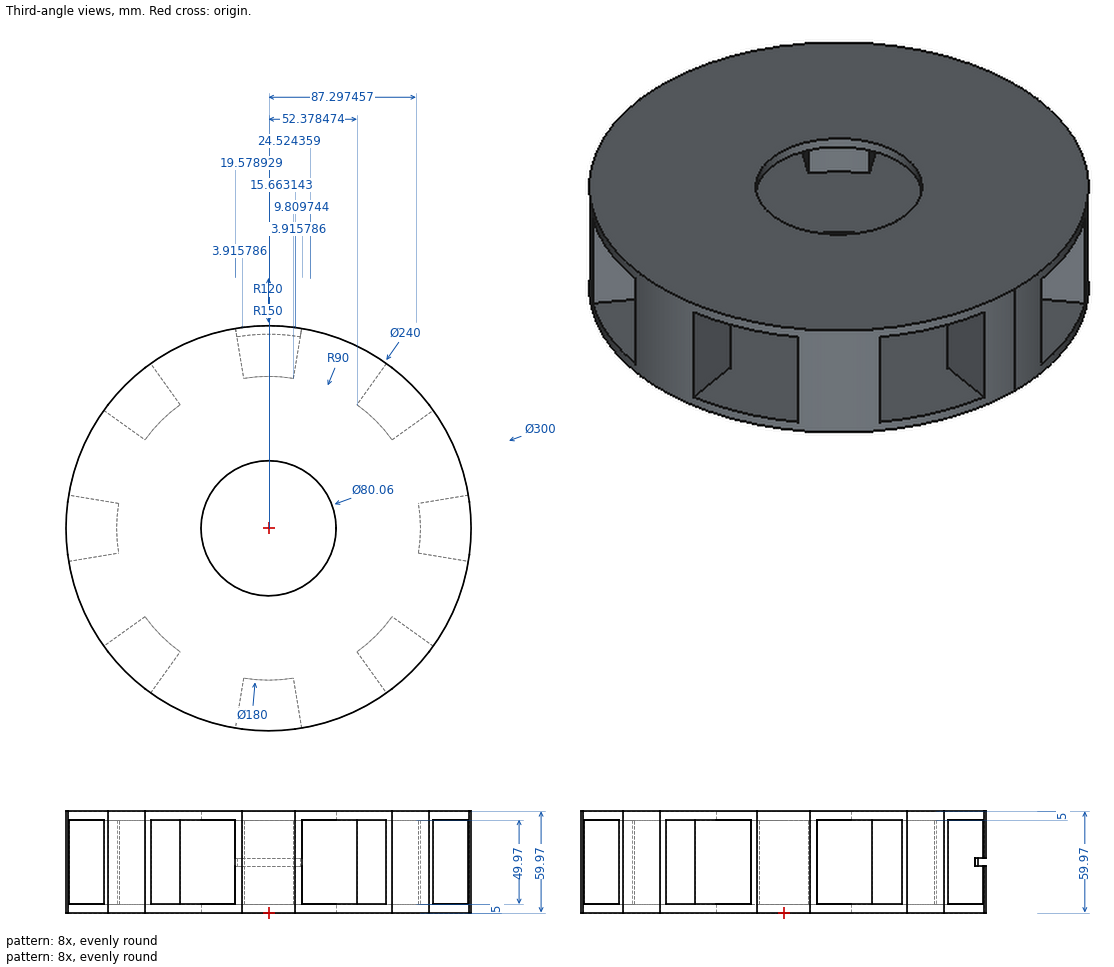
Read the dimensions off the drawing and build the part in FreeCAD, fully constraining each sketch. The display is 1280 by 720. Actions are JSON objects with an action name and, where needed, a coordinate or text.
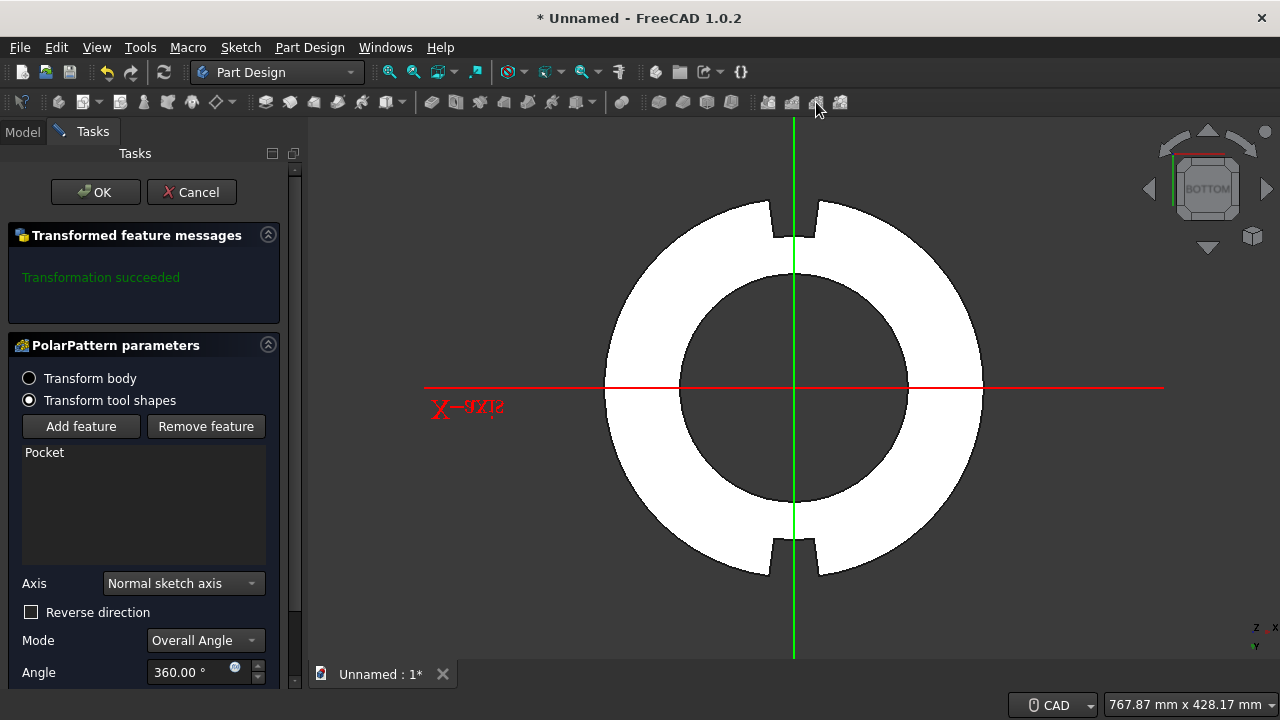
{"action": "left_click", "coordinate": [184, 584]}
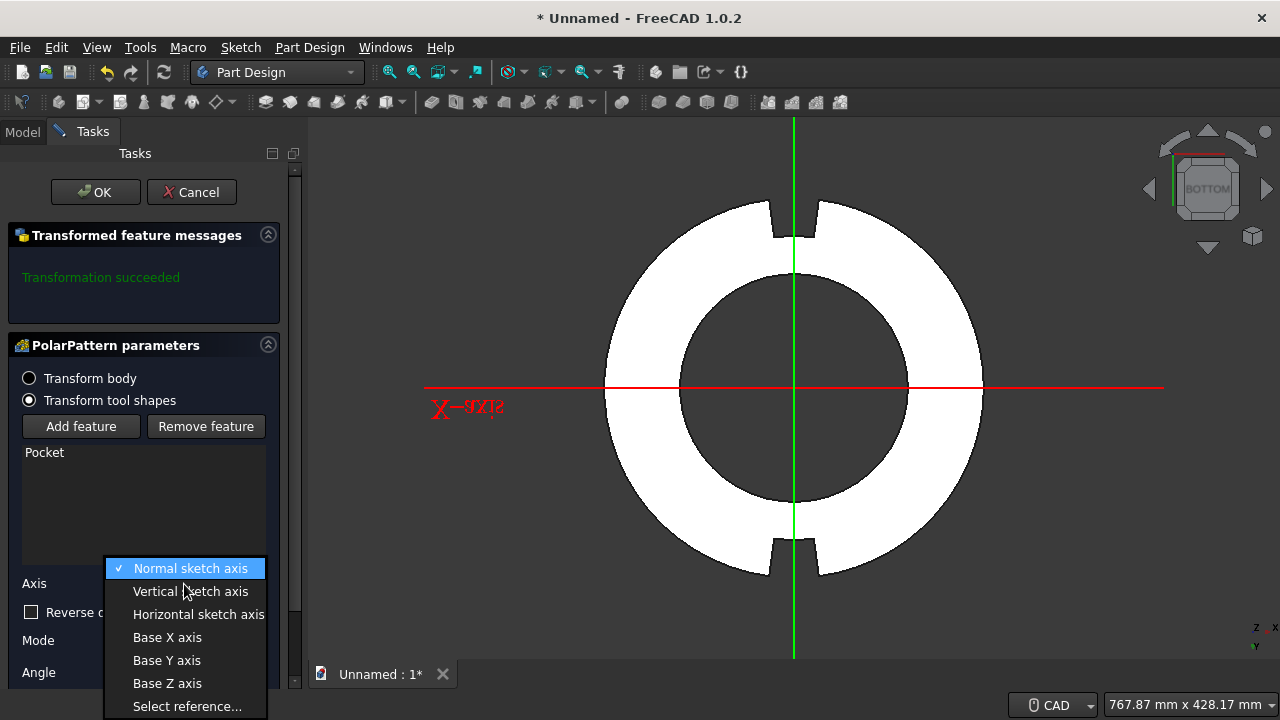
{"action": "left_click", "coordinate": [184, 684]}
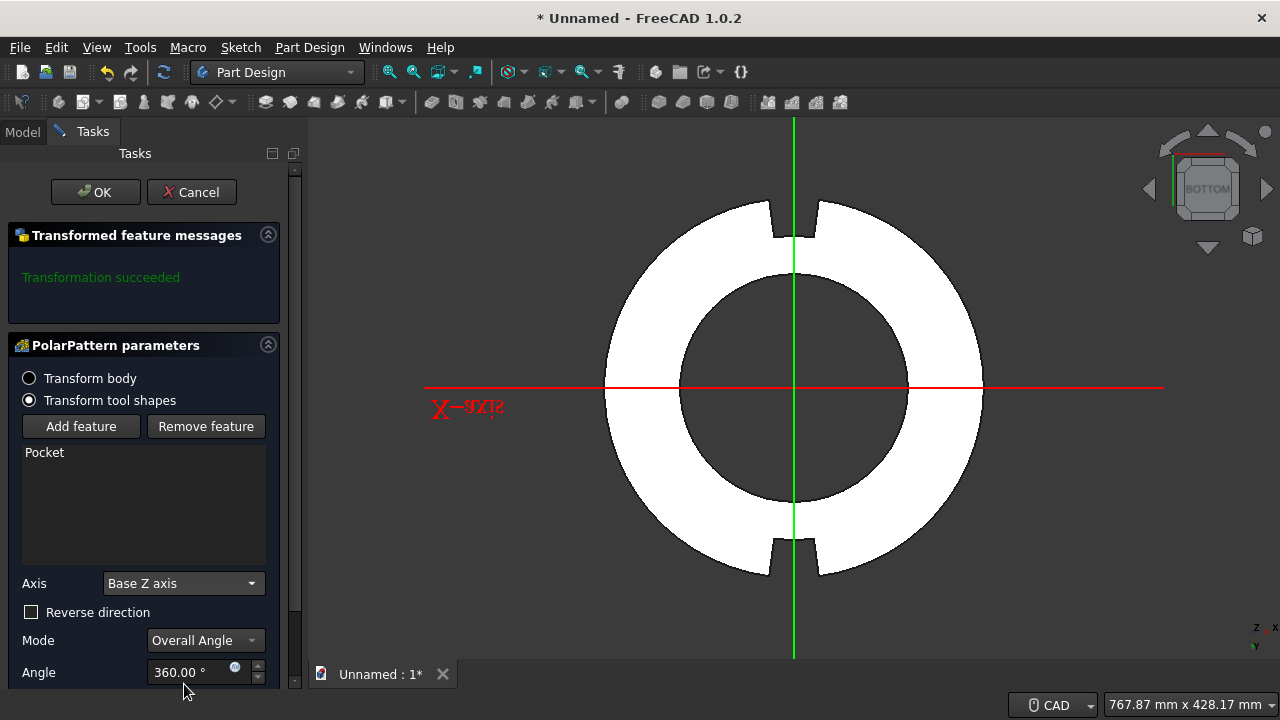
{"action": "scroll", "coordinate": [295, 426], "scroll_direction": "down", "scroll_amount": 2}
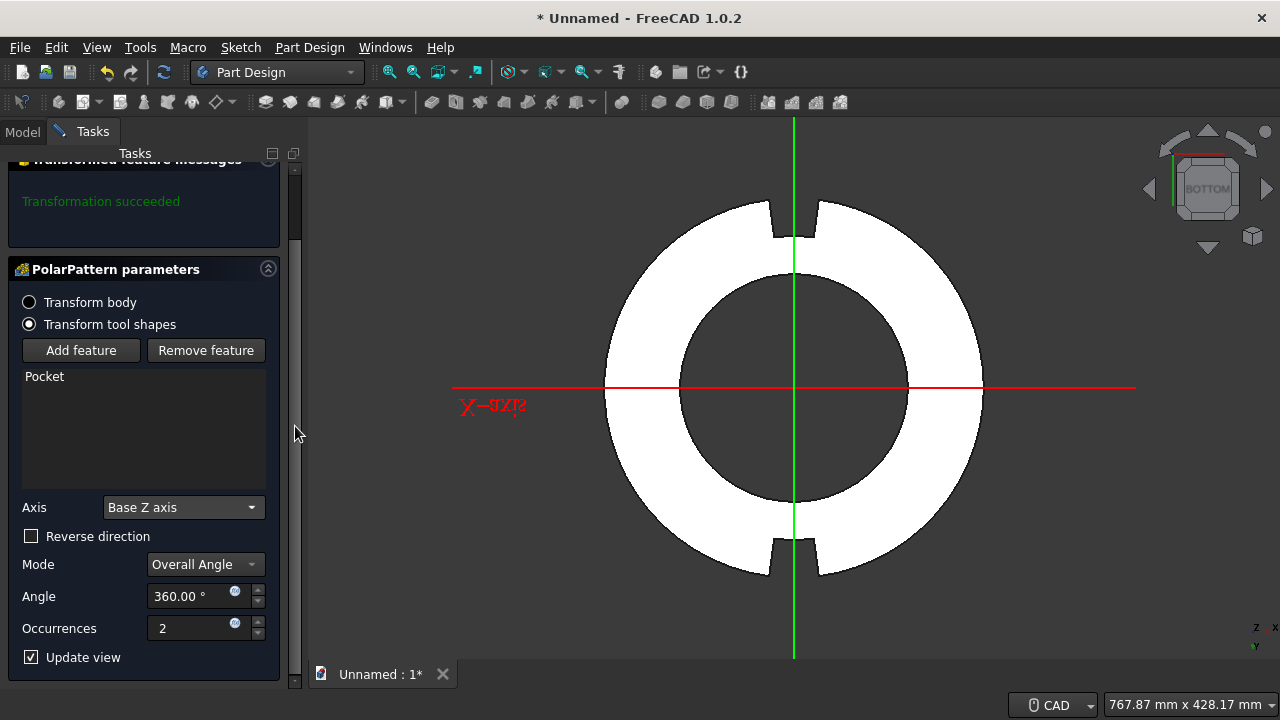
{"action": "triple_click", "coordinate": [198, 628]}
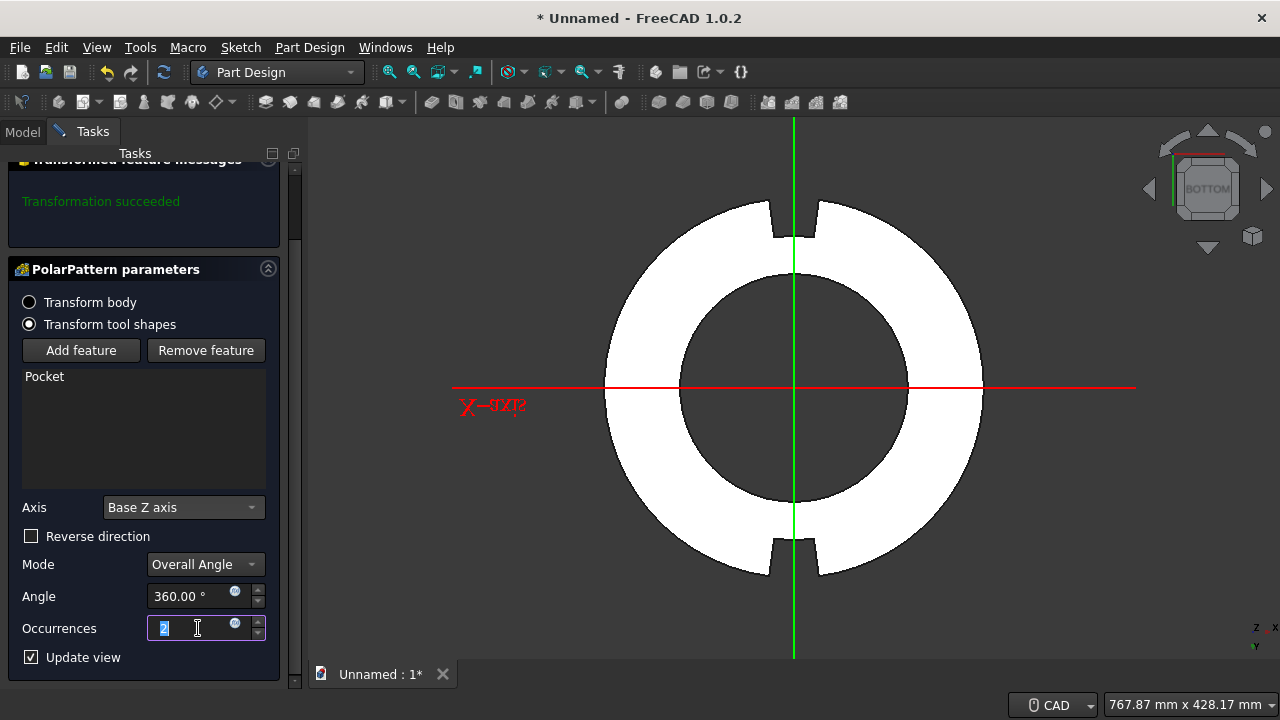
{"action": "type", "text": "8"}
{"action": "key", "text": "Tab"}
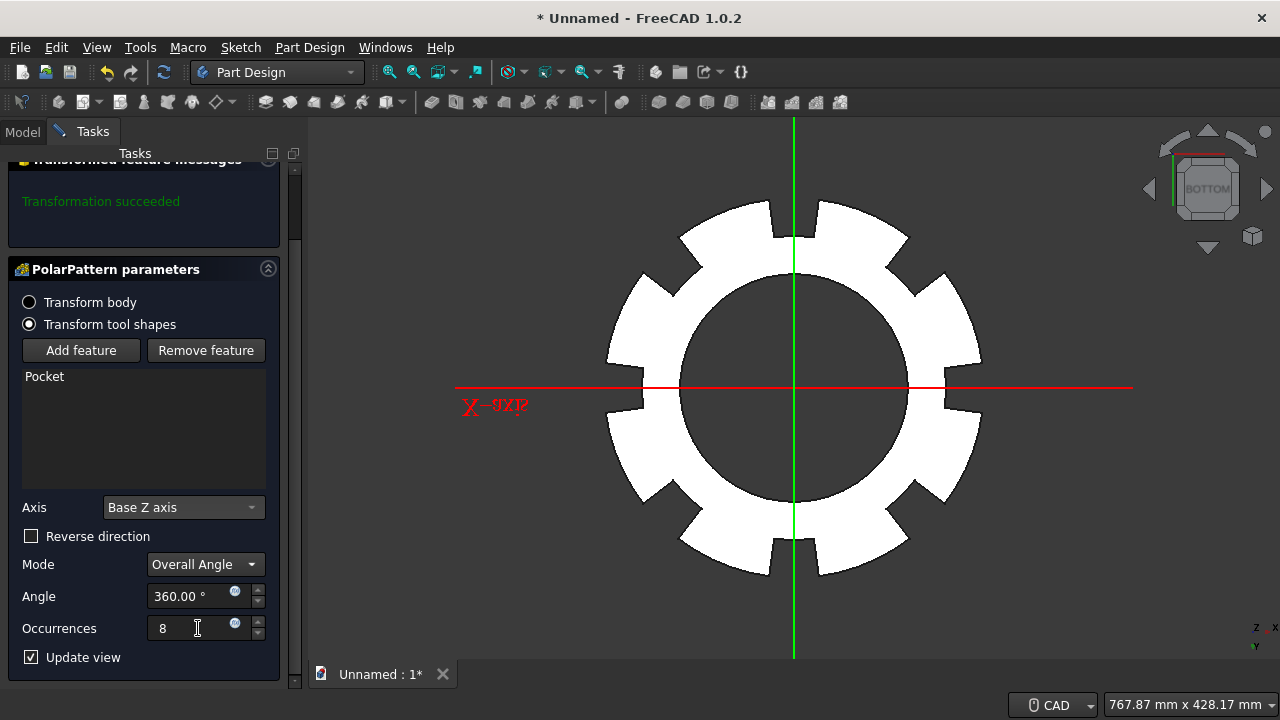
{"action": "scroll", "coordinate": [295, 426], "scroll_direction": "up", "scroll_amount": 3}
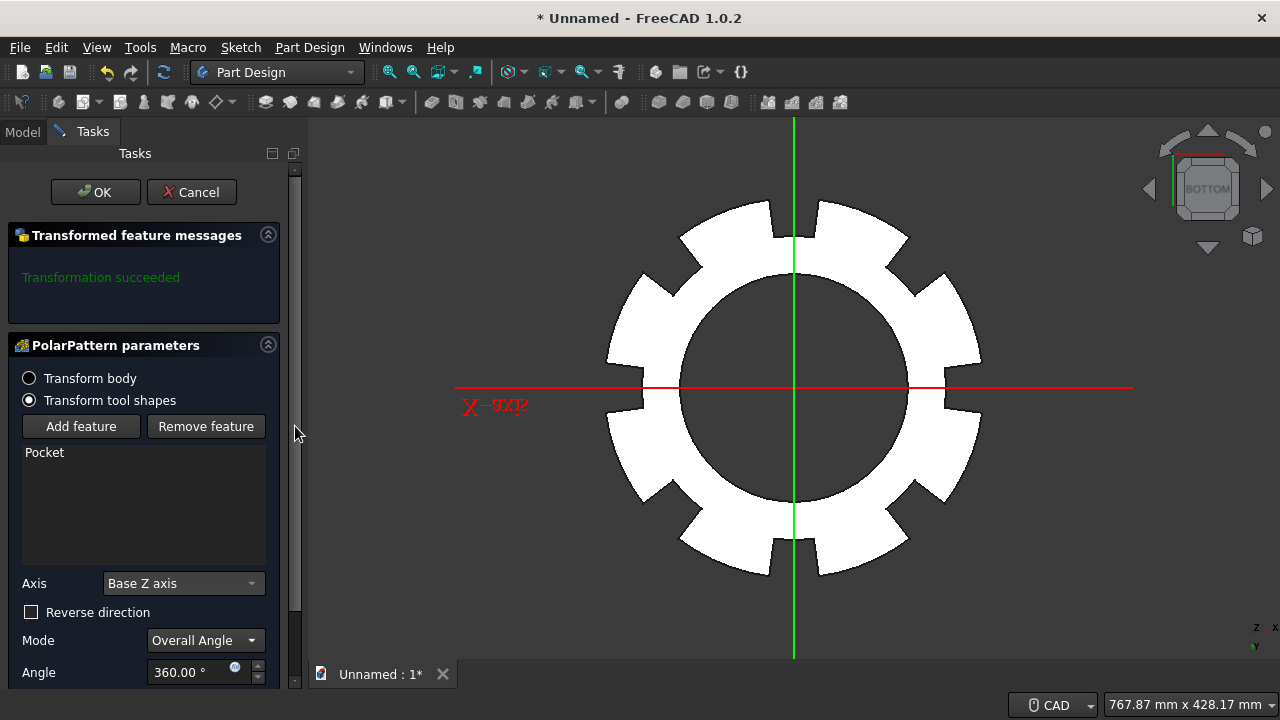
{"action": "left_click", "coordinate": [96, 192]}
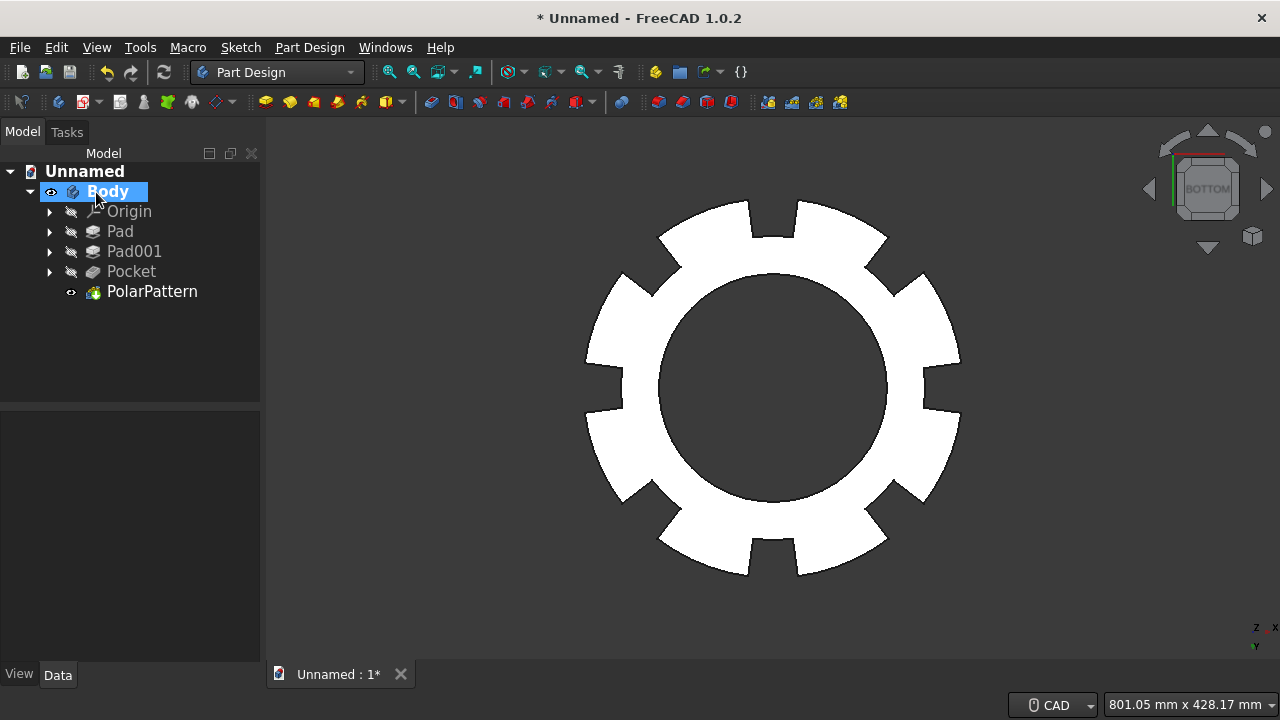
{"action": "left_click", "coordinate": [50, 212]}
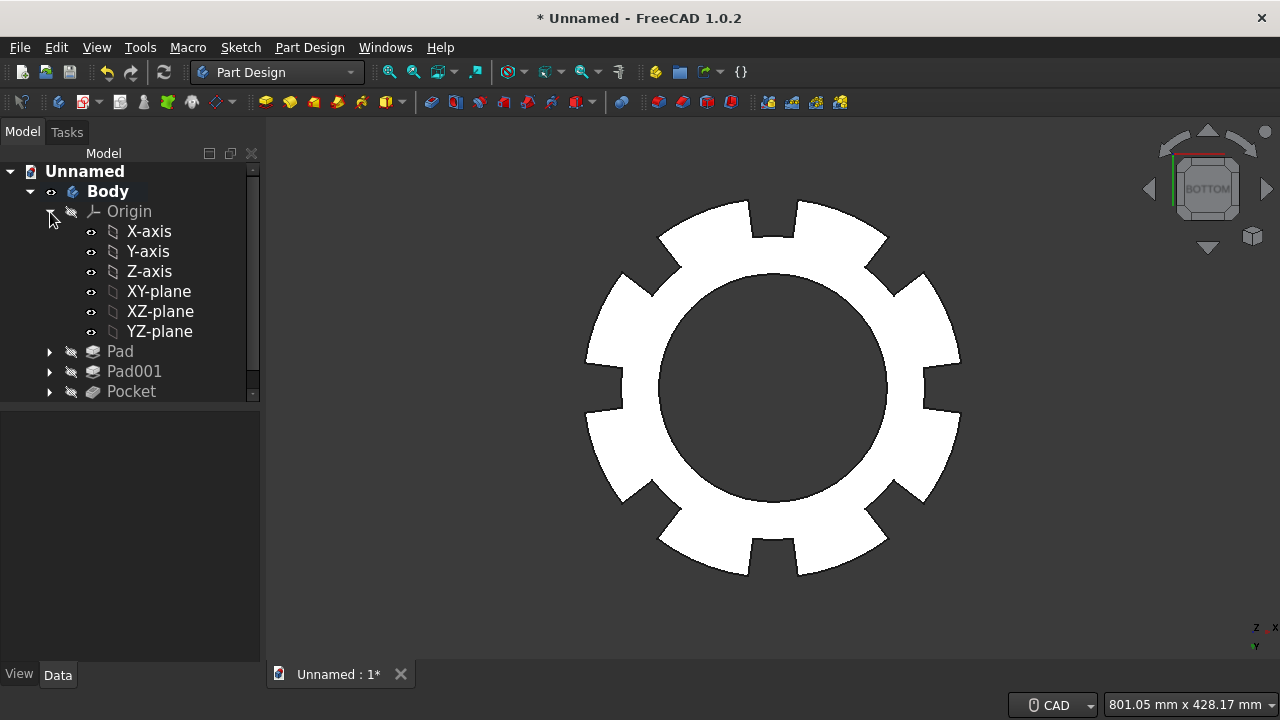
{"action": "left_click", "coordinate": [136, 292]}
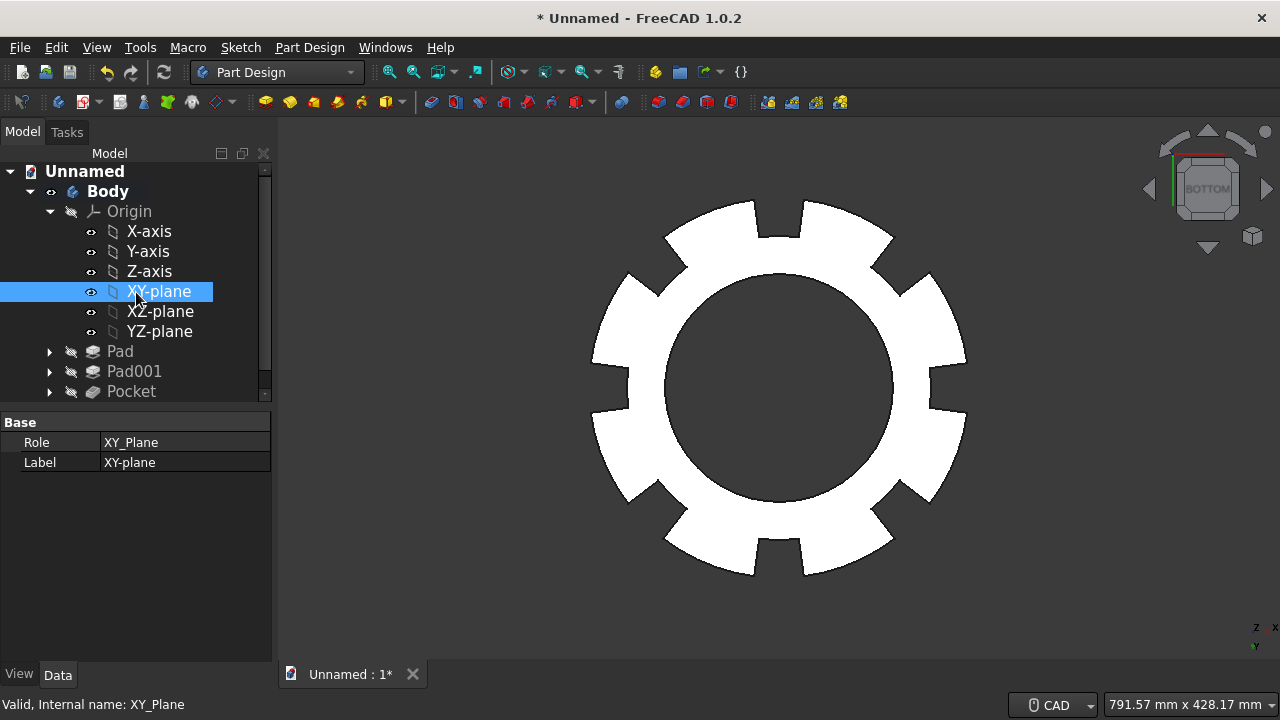
{"action": "left_click", "coordinate": [216, 102]}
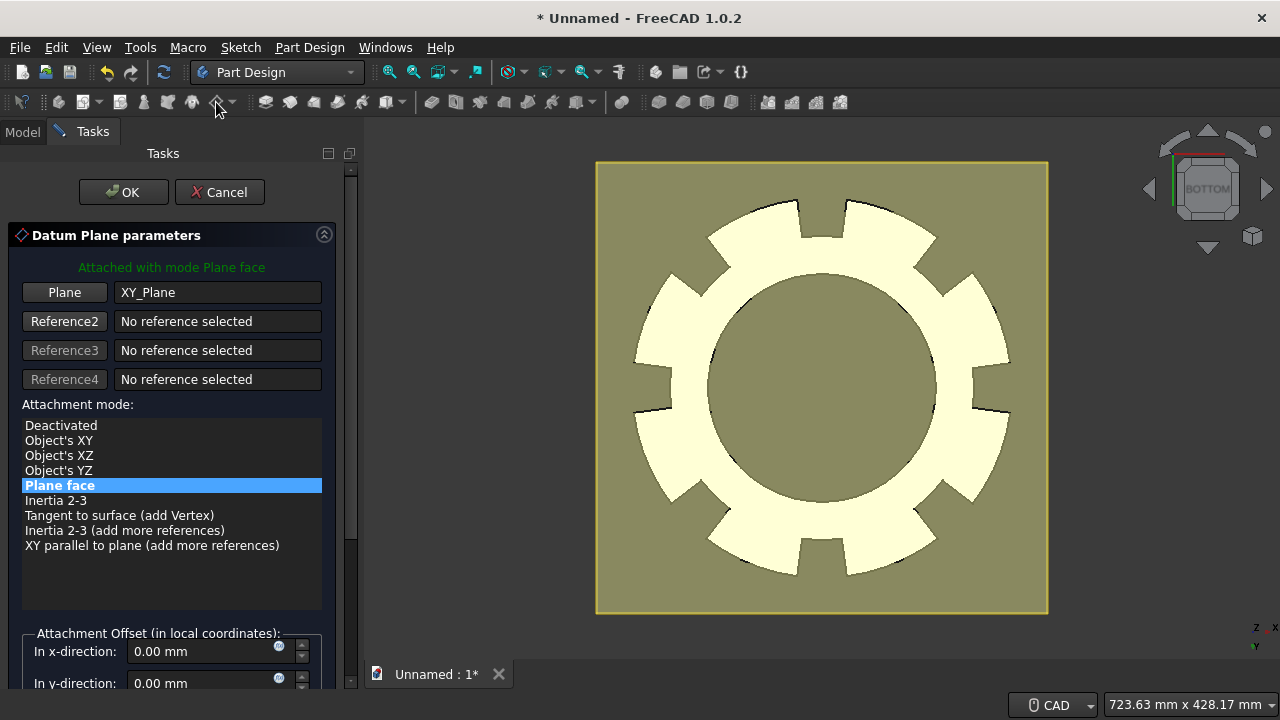
{"action": "scroll", "coordinate": [351, 426], "scroll_direction": "down", "scroll_amount": 2}